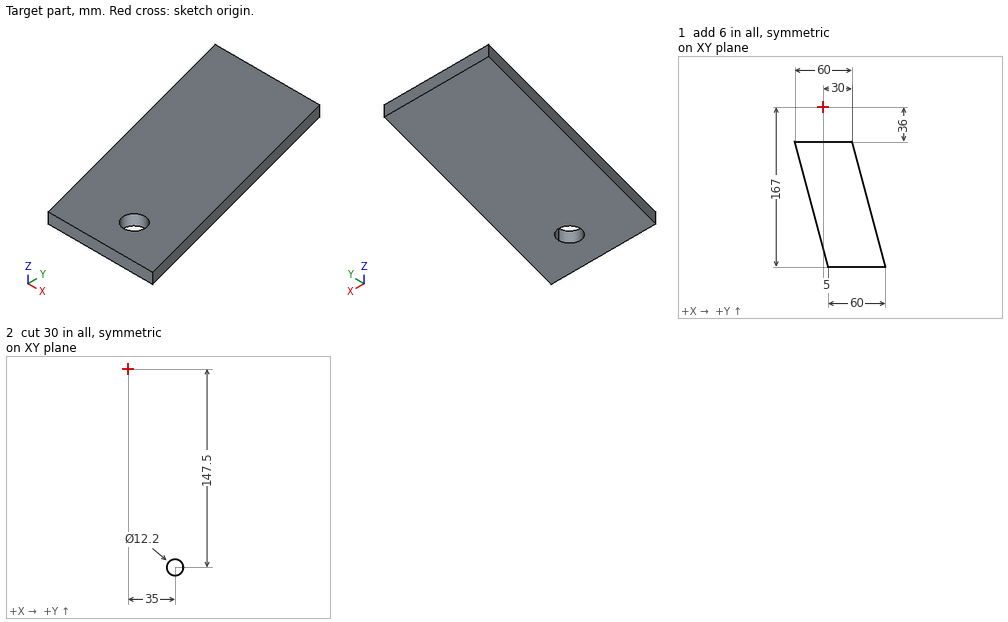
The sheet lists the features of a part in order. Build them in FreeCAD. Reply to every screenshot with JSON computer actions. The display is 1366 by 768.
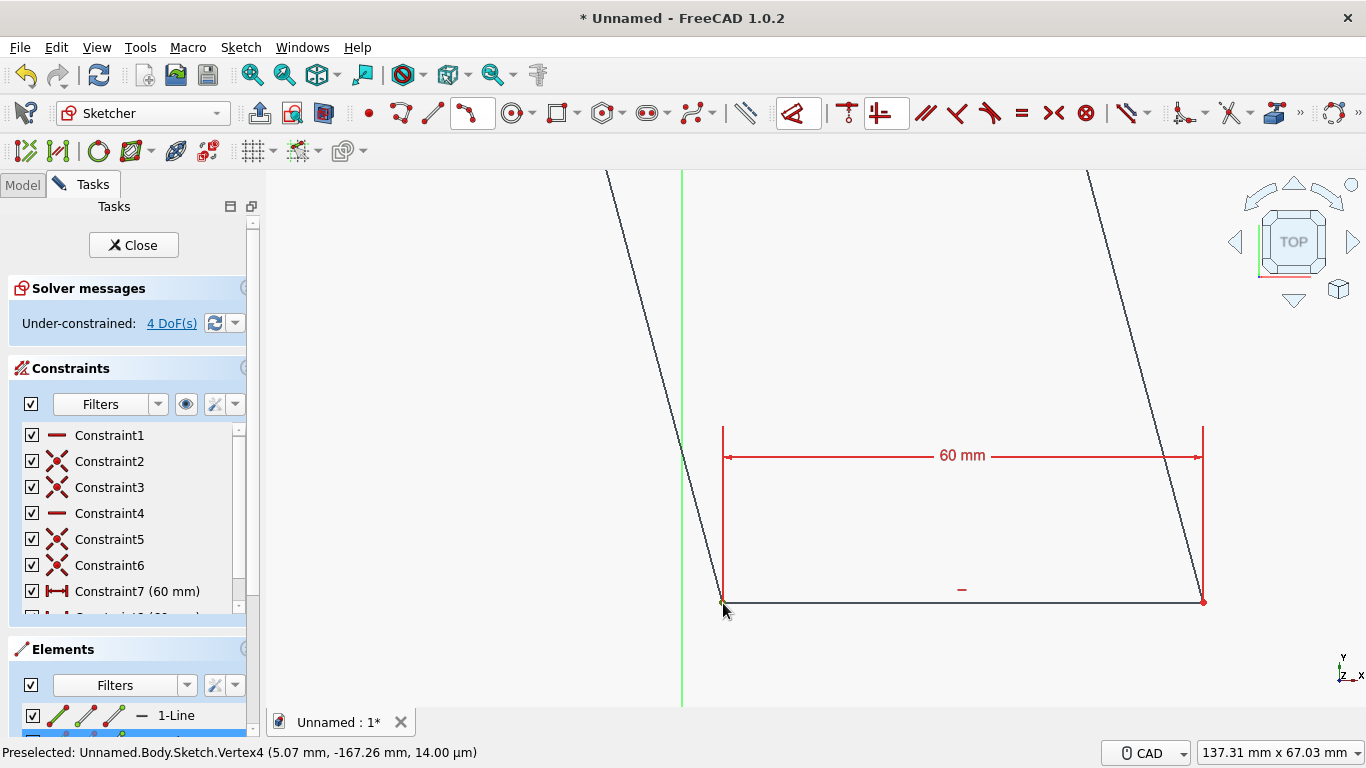
{"action": "left_click", "coordinate": [816, 114]}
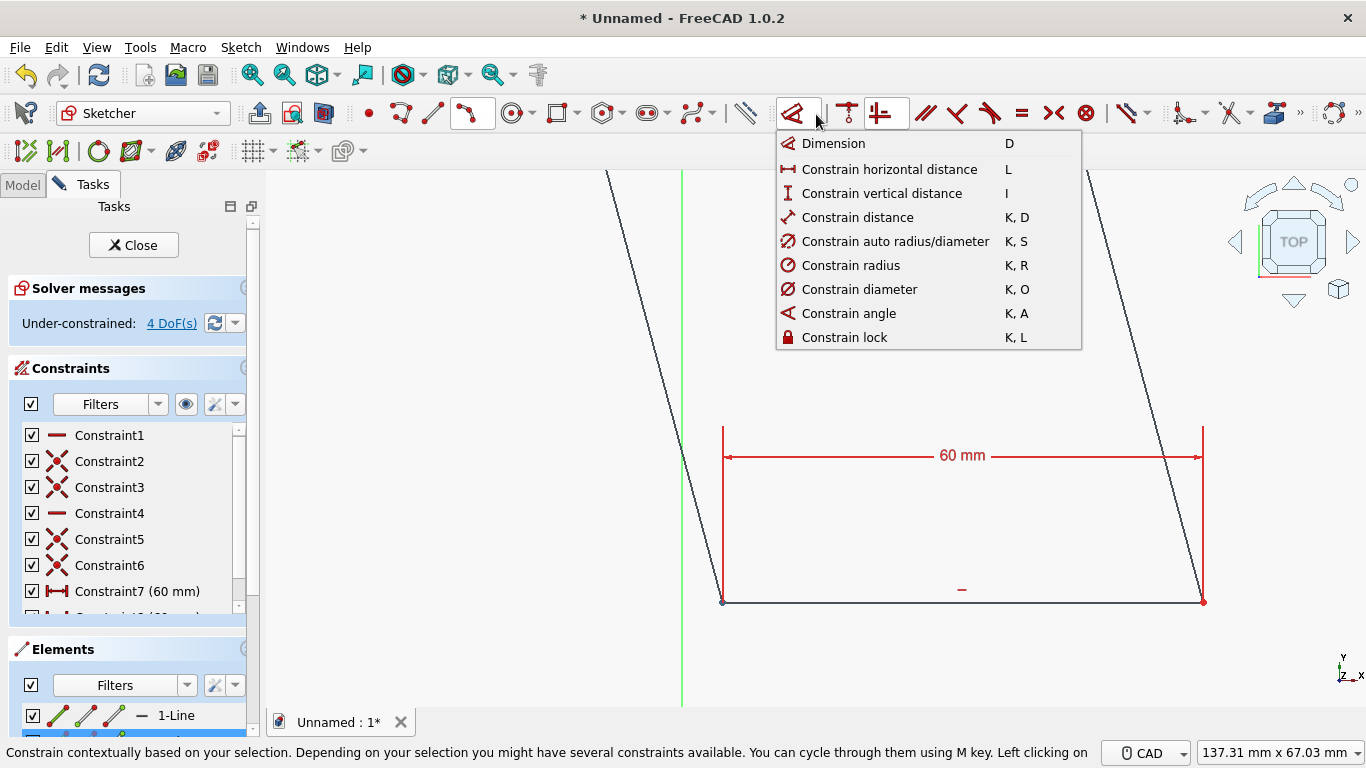
{"action": "left_click", "coordinate": [929, 169]}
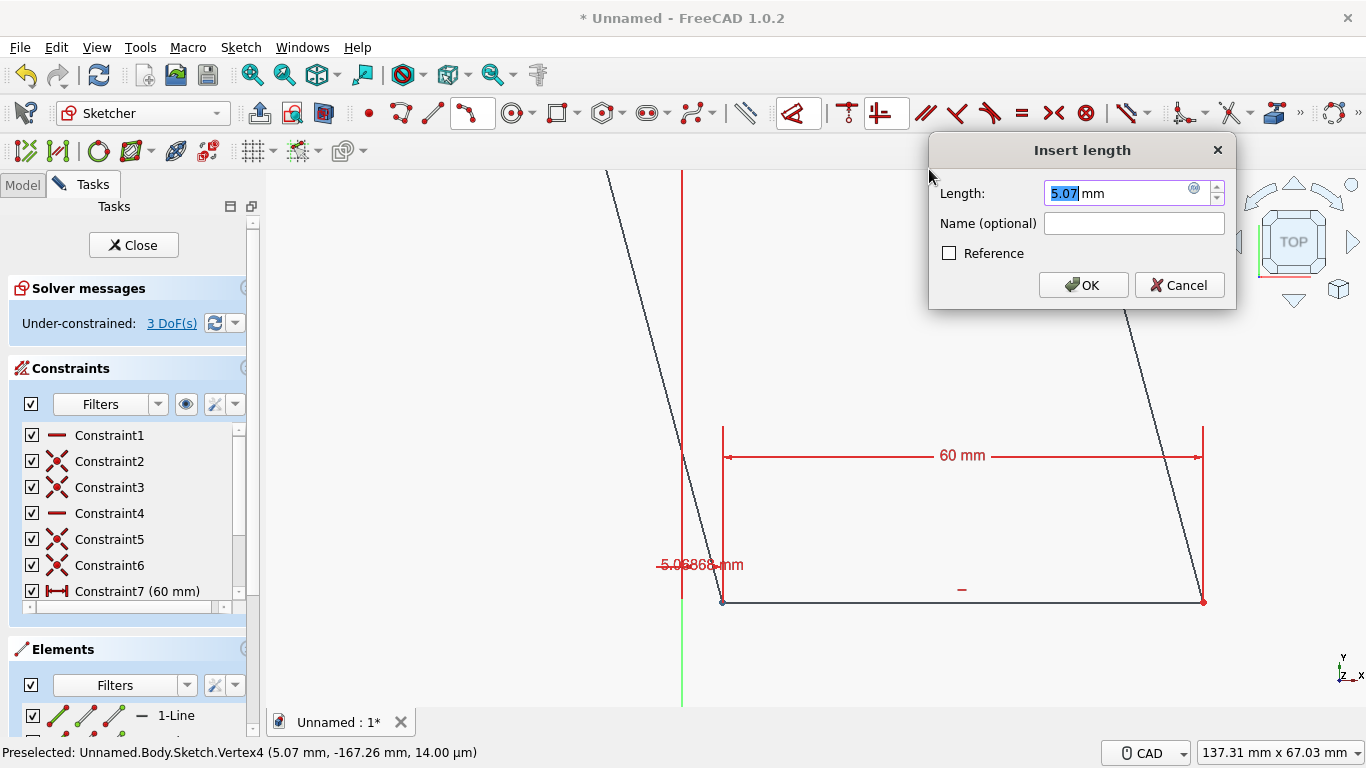
{"action": "type", "text": "5"}
{"action": "key", "text": "Return"}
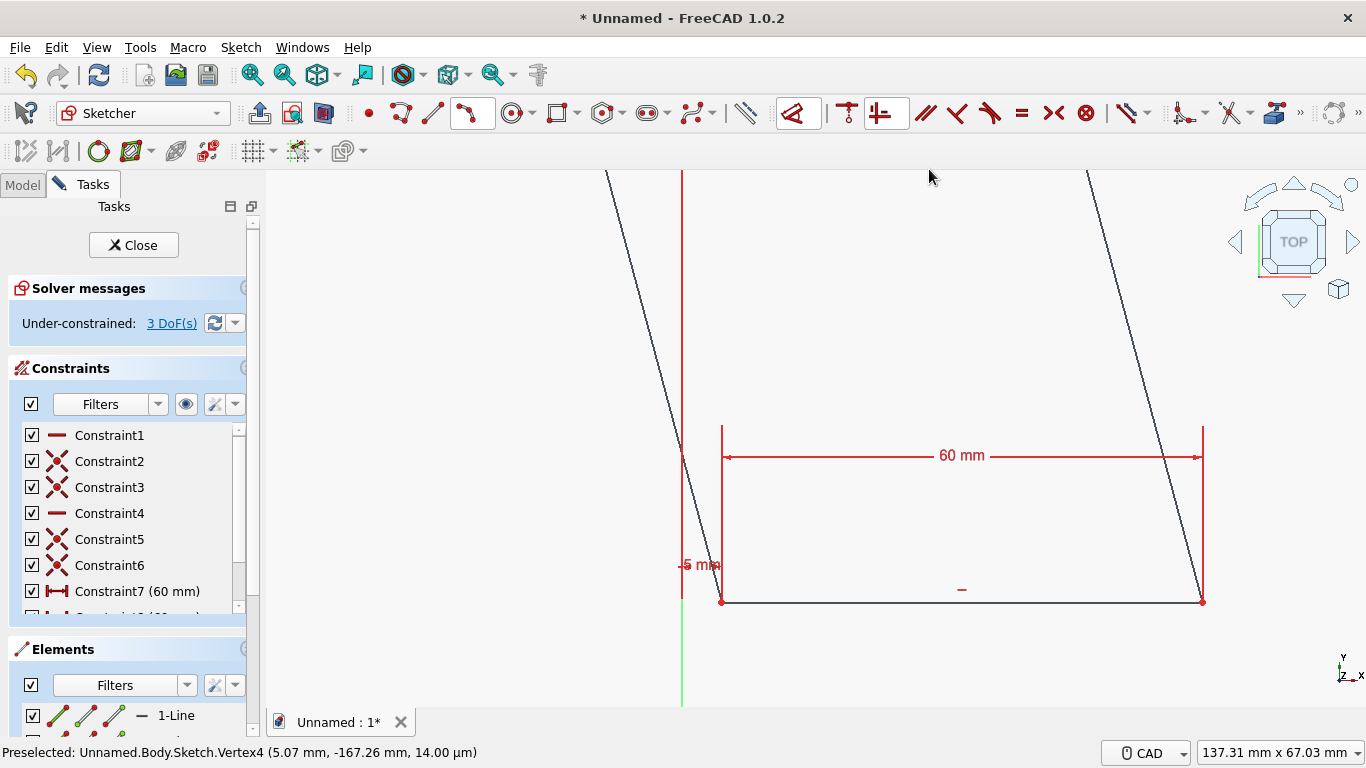
{"action": "scroll", "coordinate": [723, 604], "scroll_direction": "down", "scroll_amount": 7}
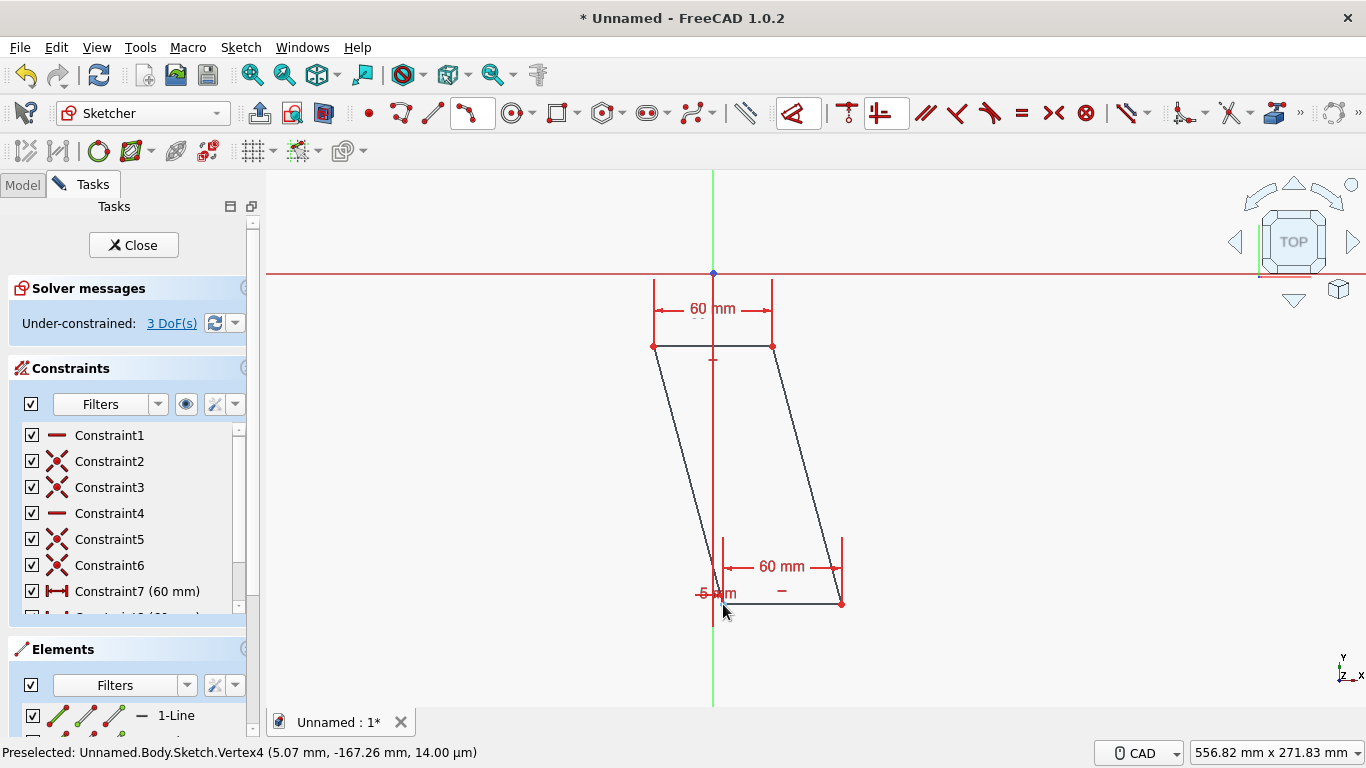
{"action": "left_click", "coordinate": [772, 346]}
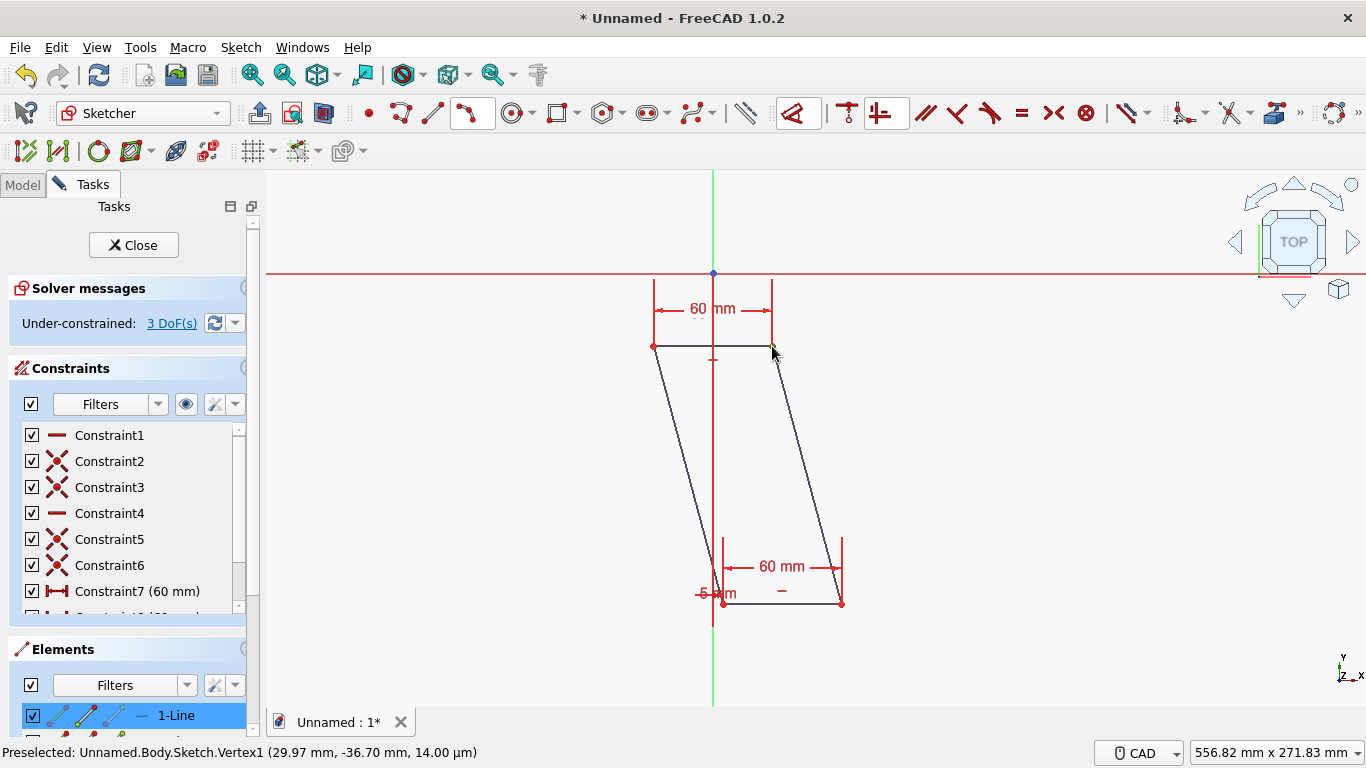
{"action": "left_click", "coordinate": [816, 114]}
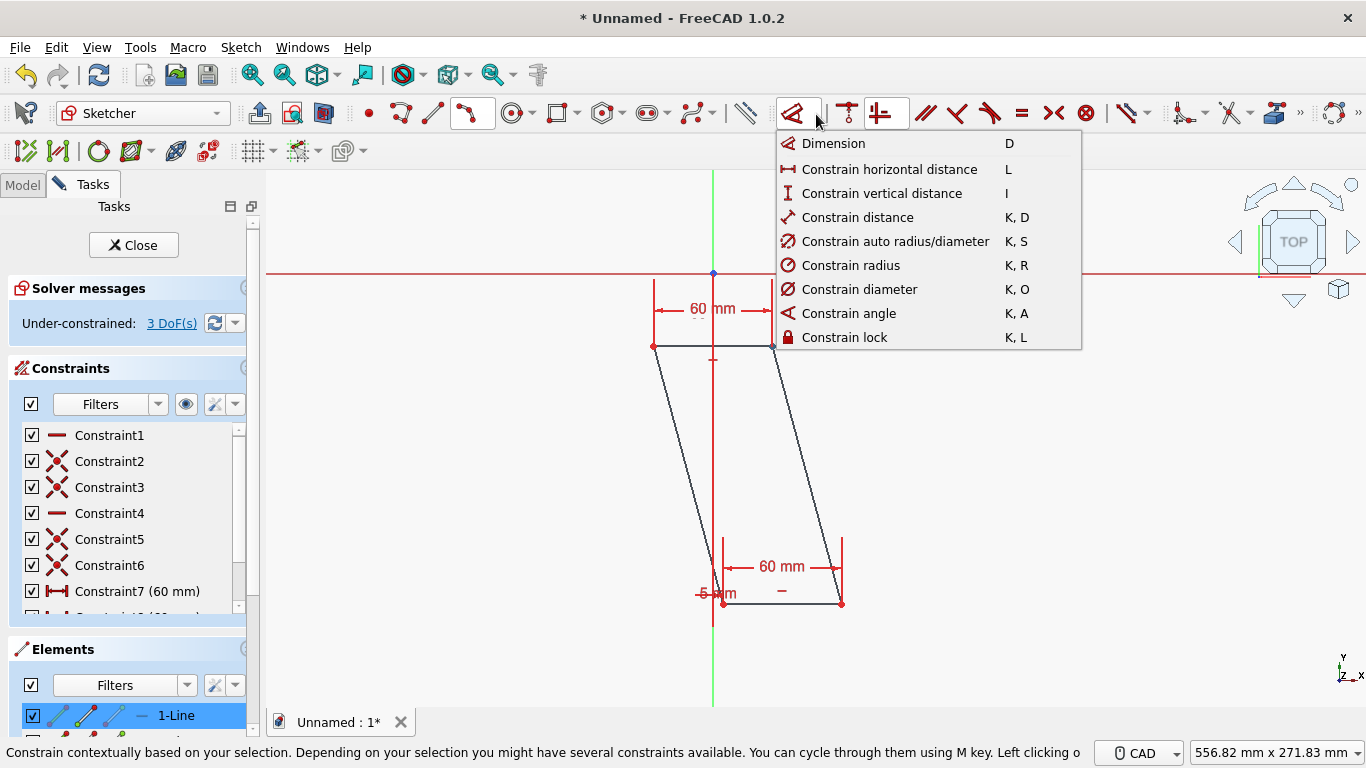
{"action": "left_click", "coordinate": [929, 169]}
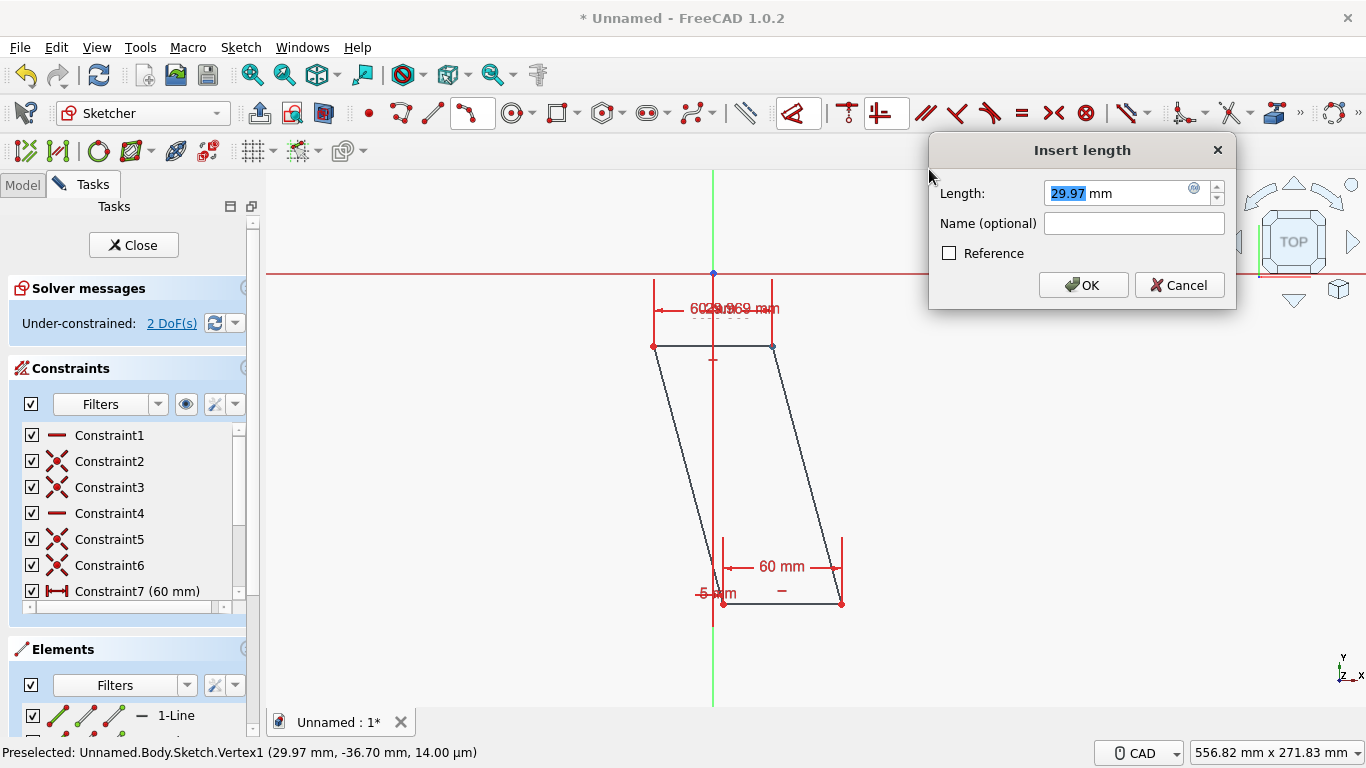
{"action": "type", "text": "30"}
{"action": "key", "text": "Return"}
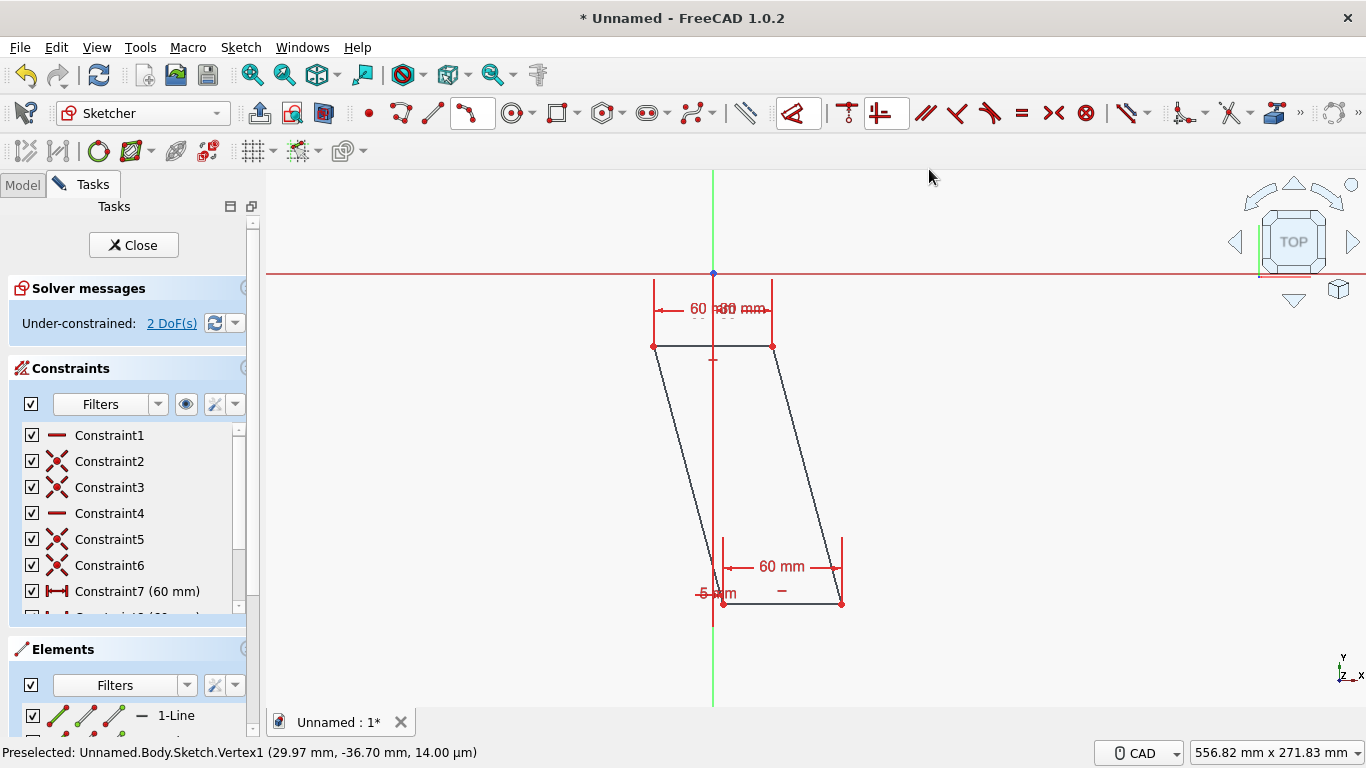
{"action": "left_click", "coordinate": [772, 346]}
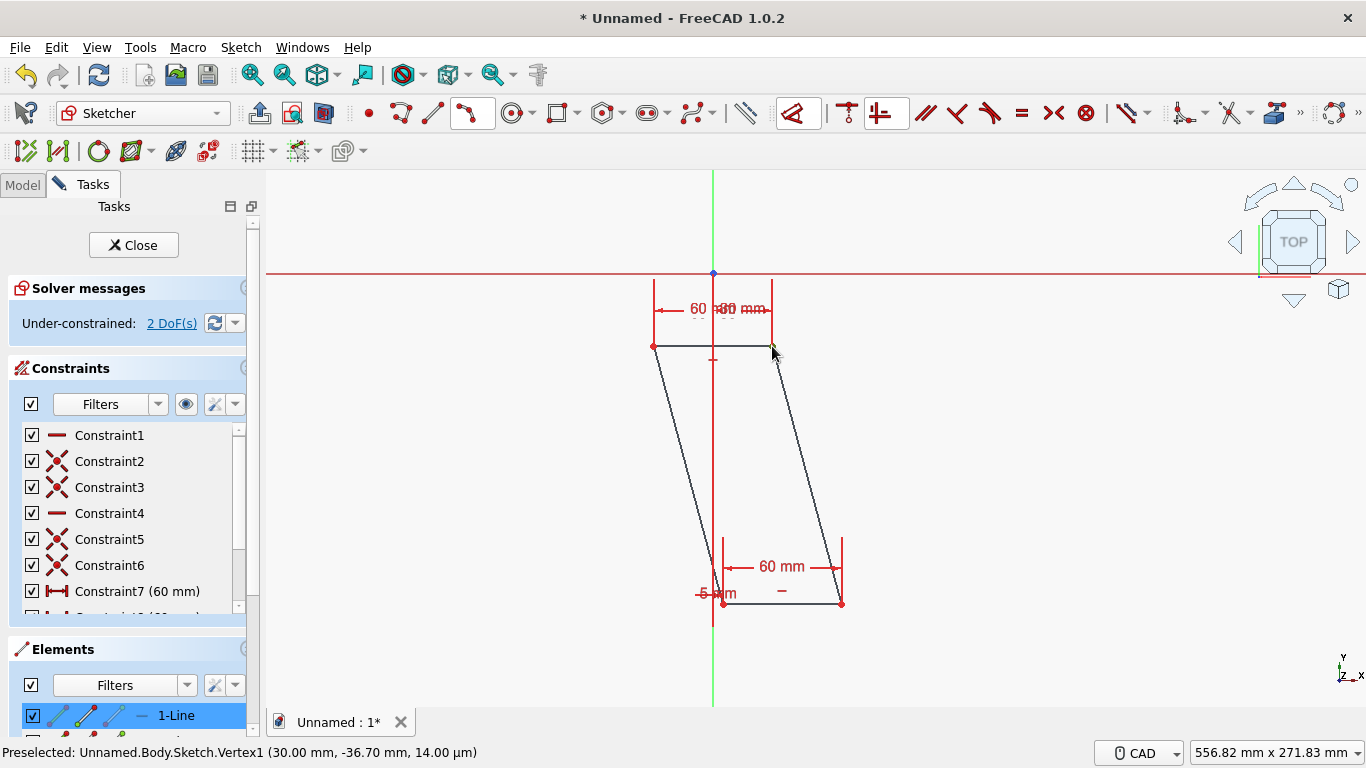
{"action": "left_click", "coordinate": [816, 114]}